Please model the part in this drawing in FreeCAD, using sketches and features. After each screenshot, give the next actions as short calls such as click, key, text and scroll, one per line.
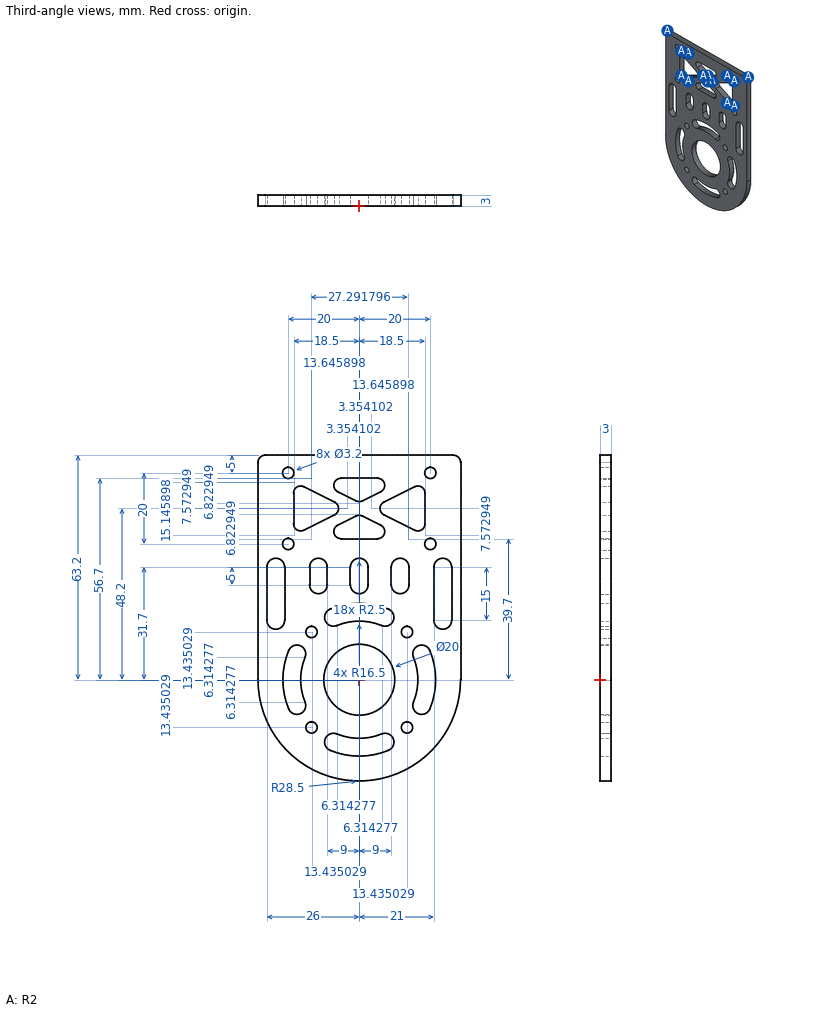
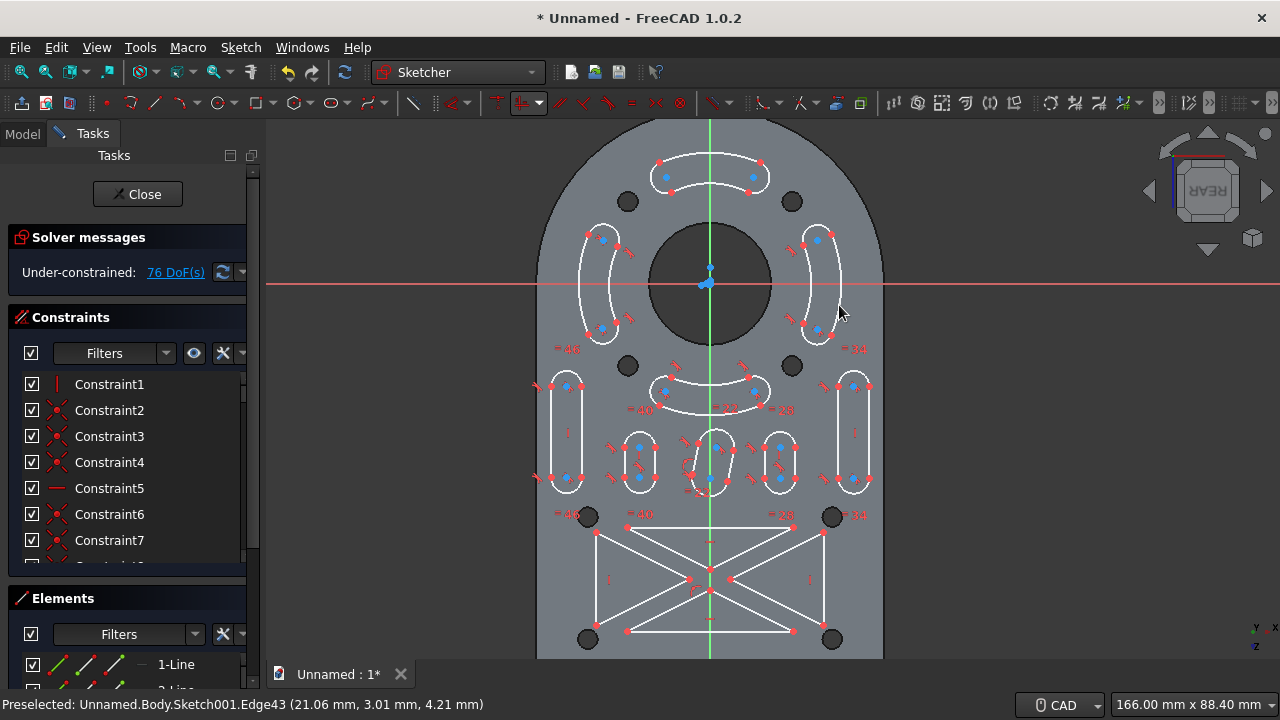
click(839, 305)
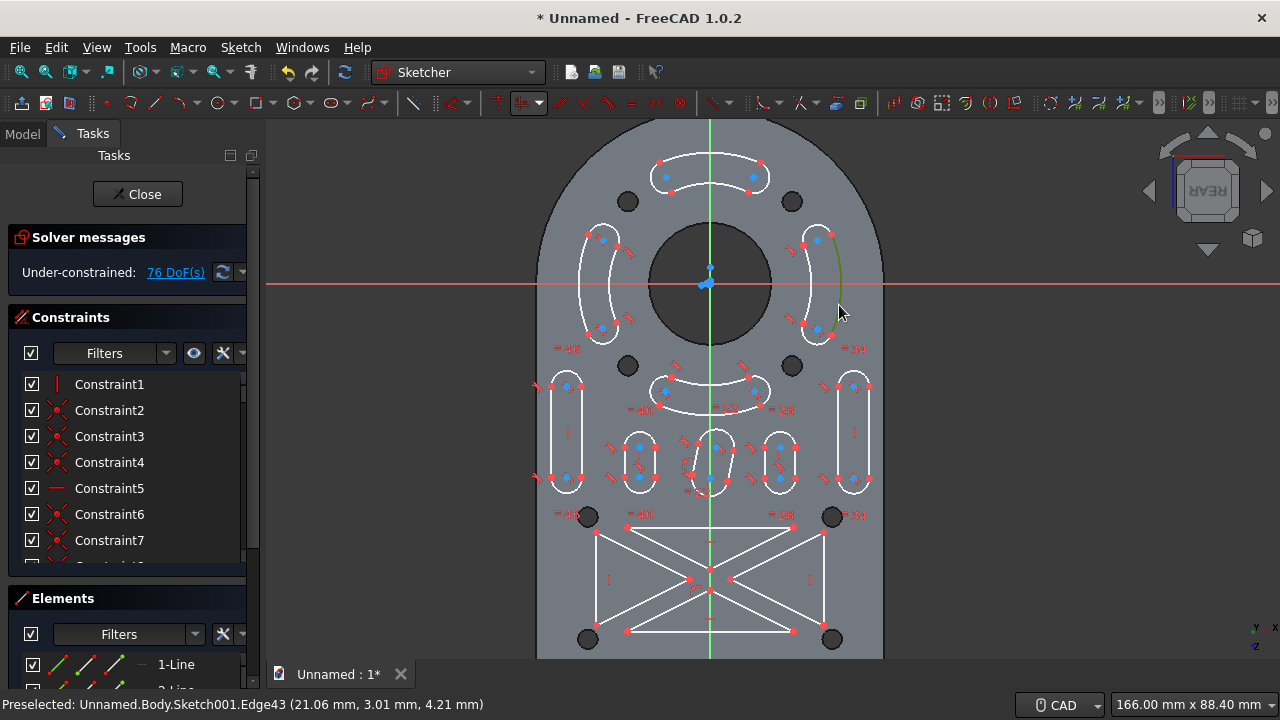
click(821, 225)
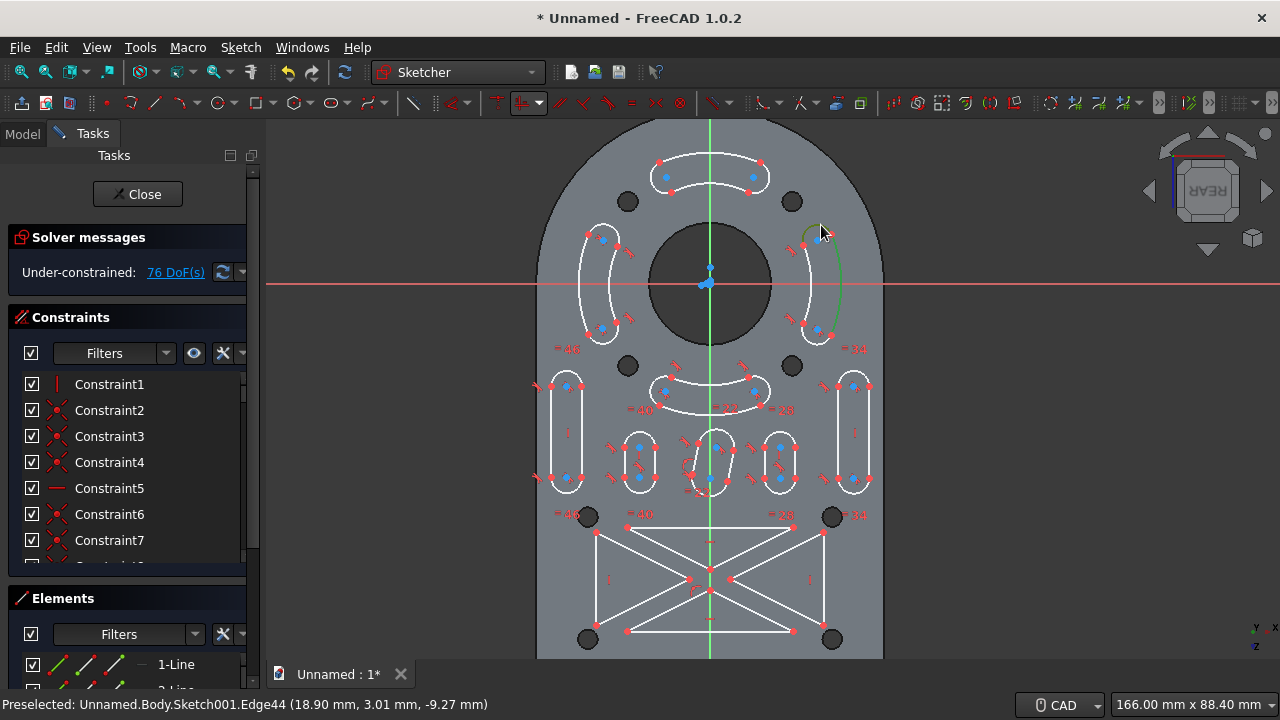
key(t)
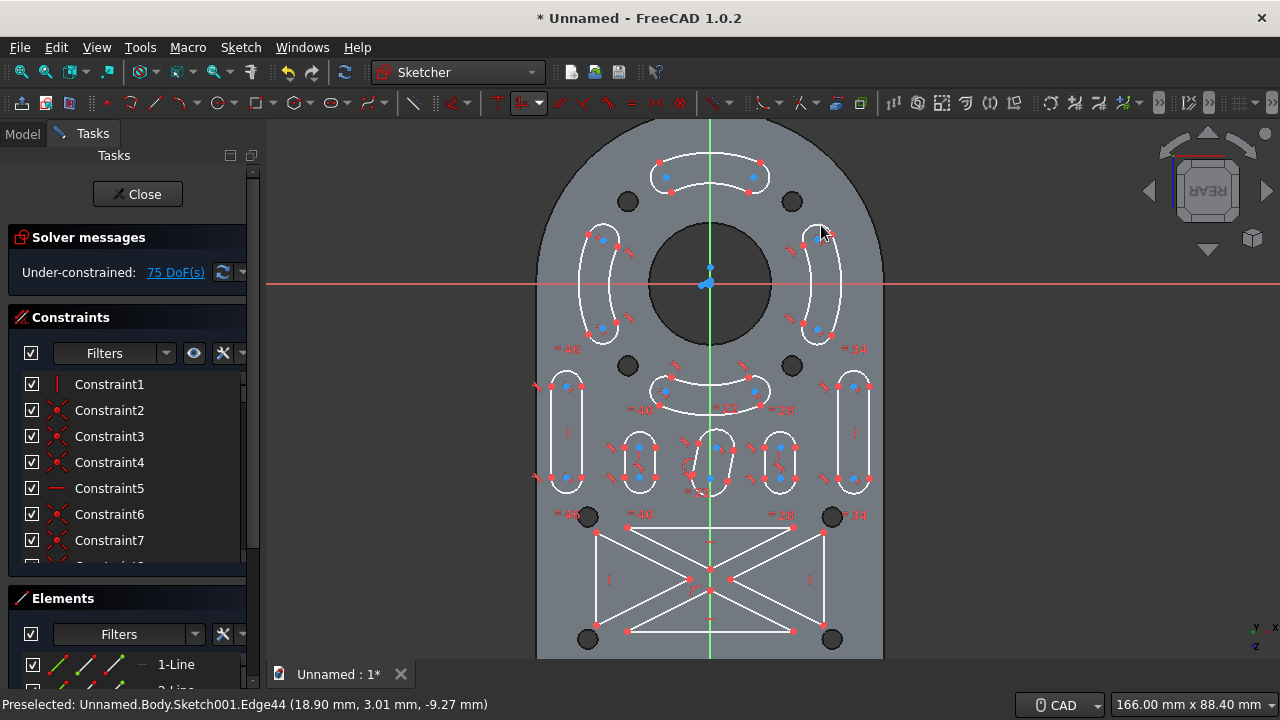
click(726, 185)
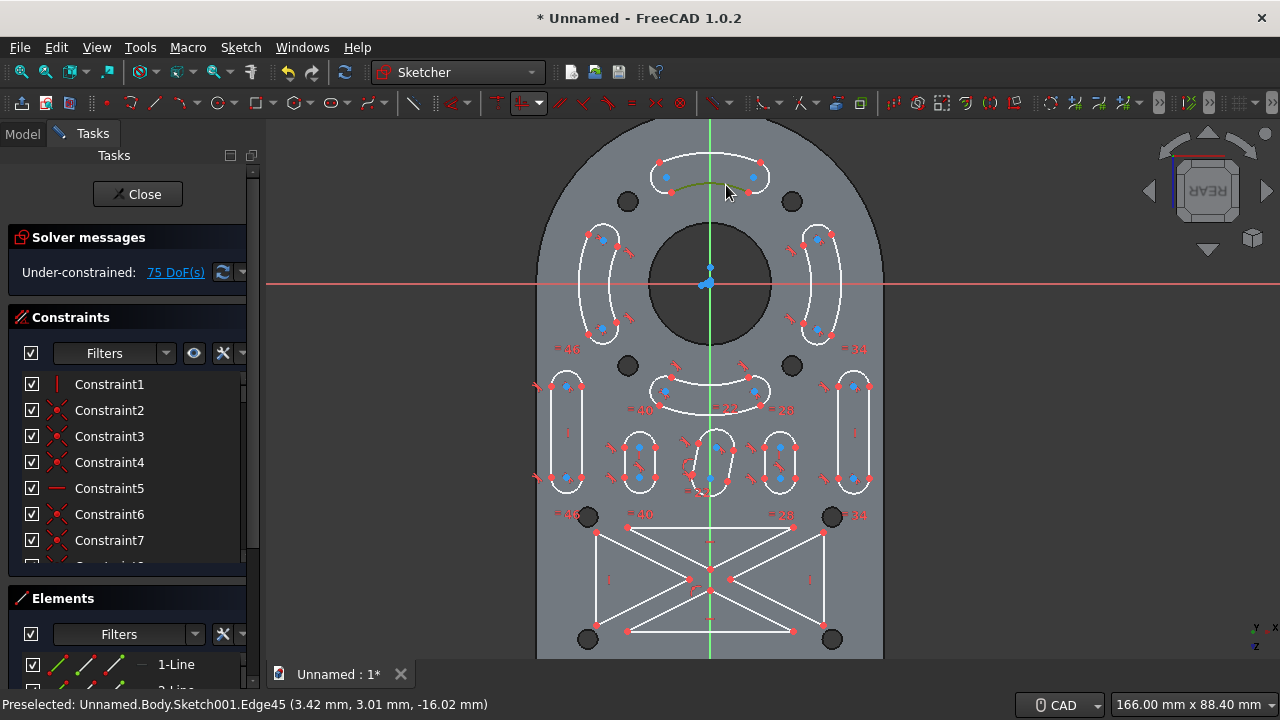
click(763, 190)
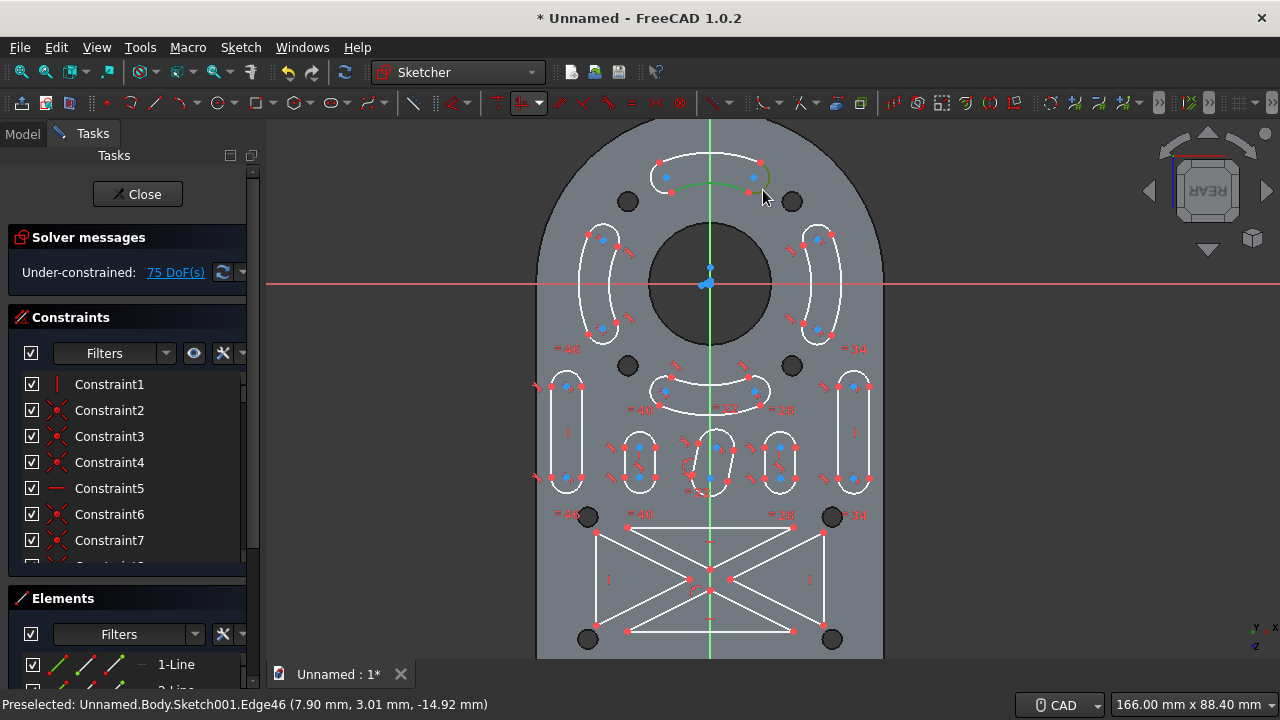
click(608, 104)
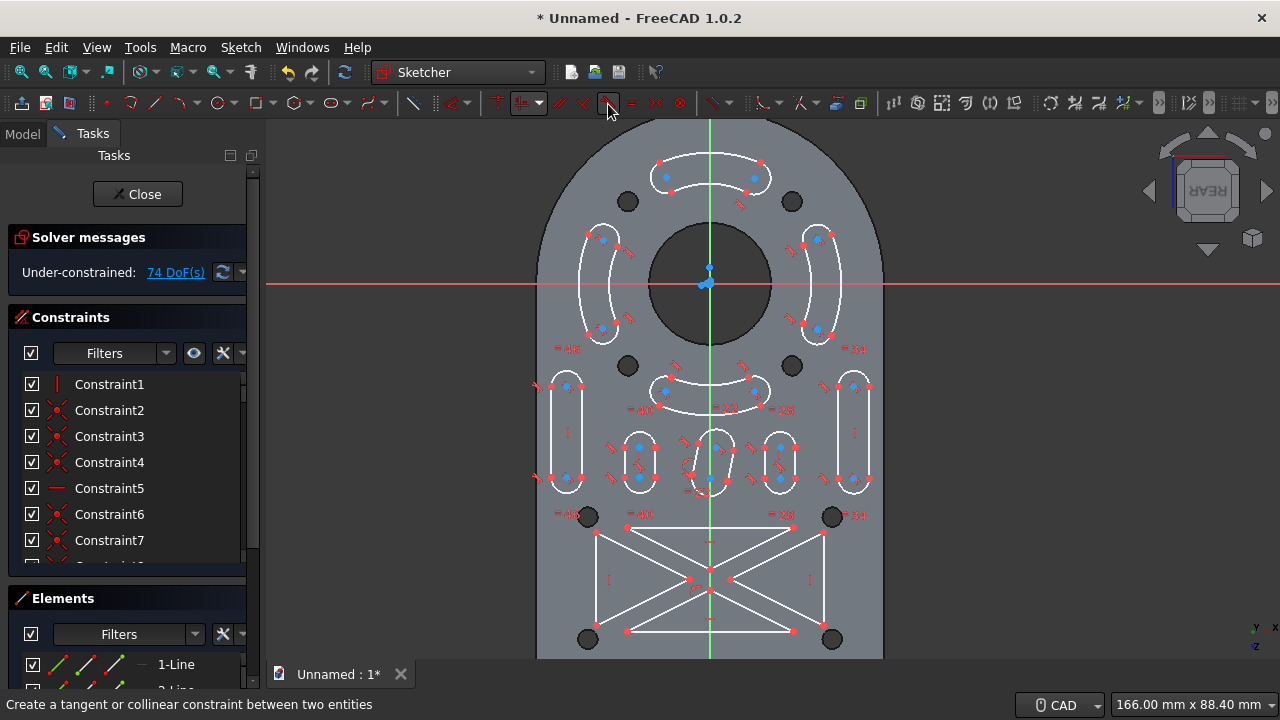
click(725, 185)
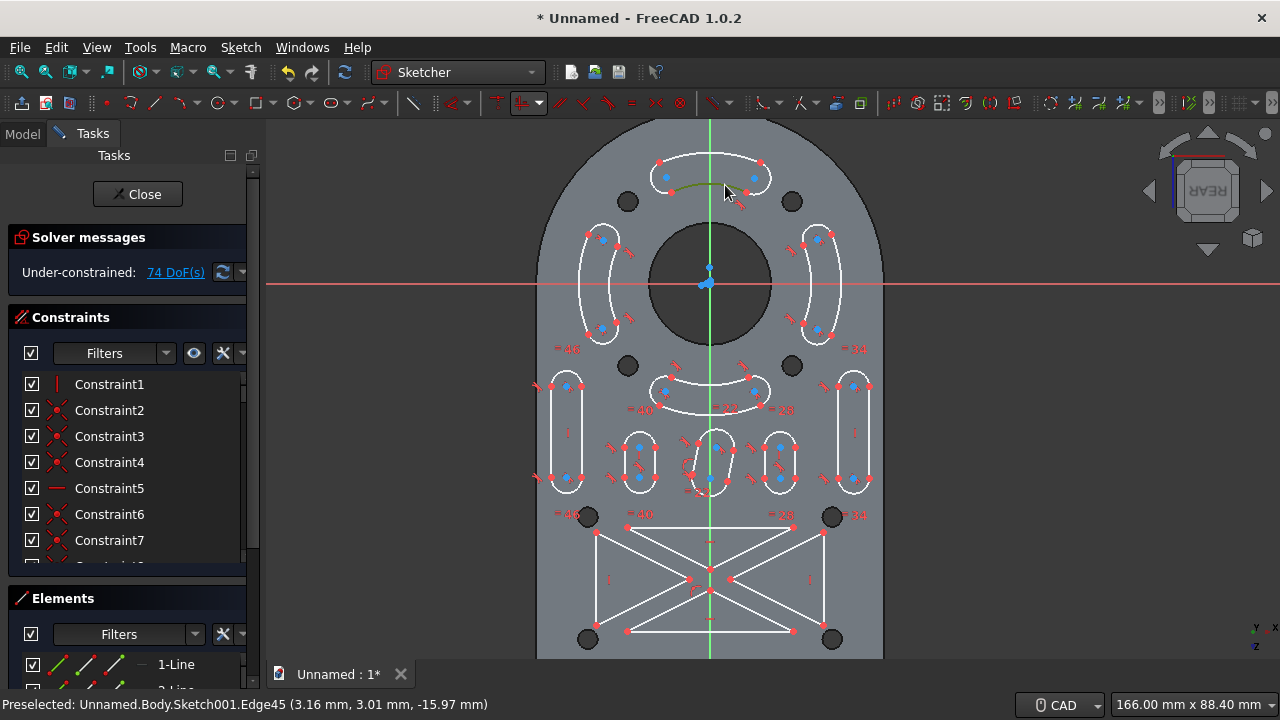
click(651, 174)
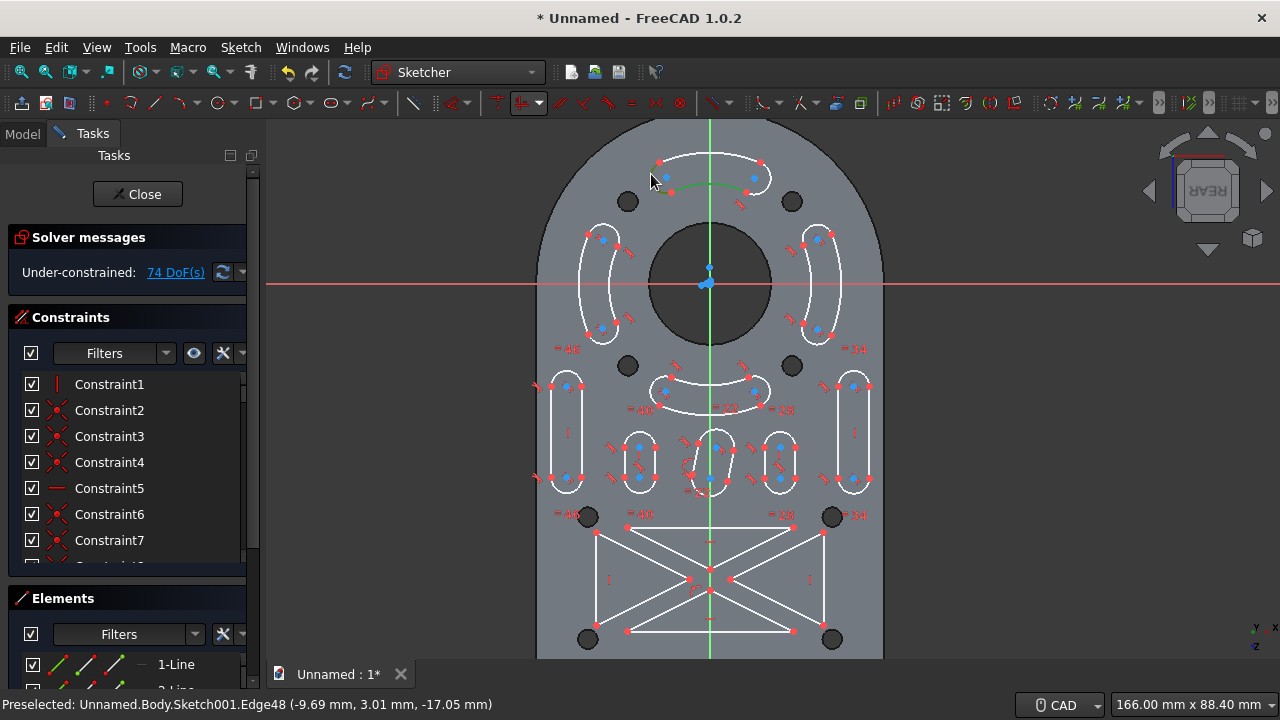
click(608, 104)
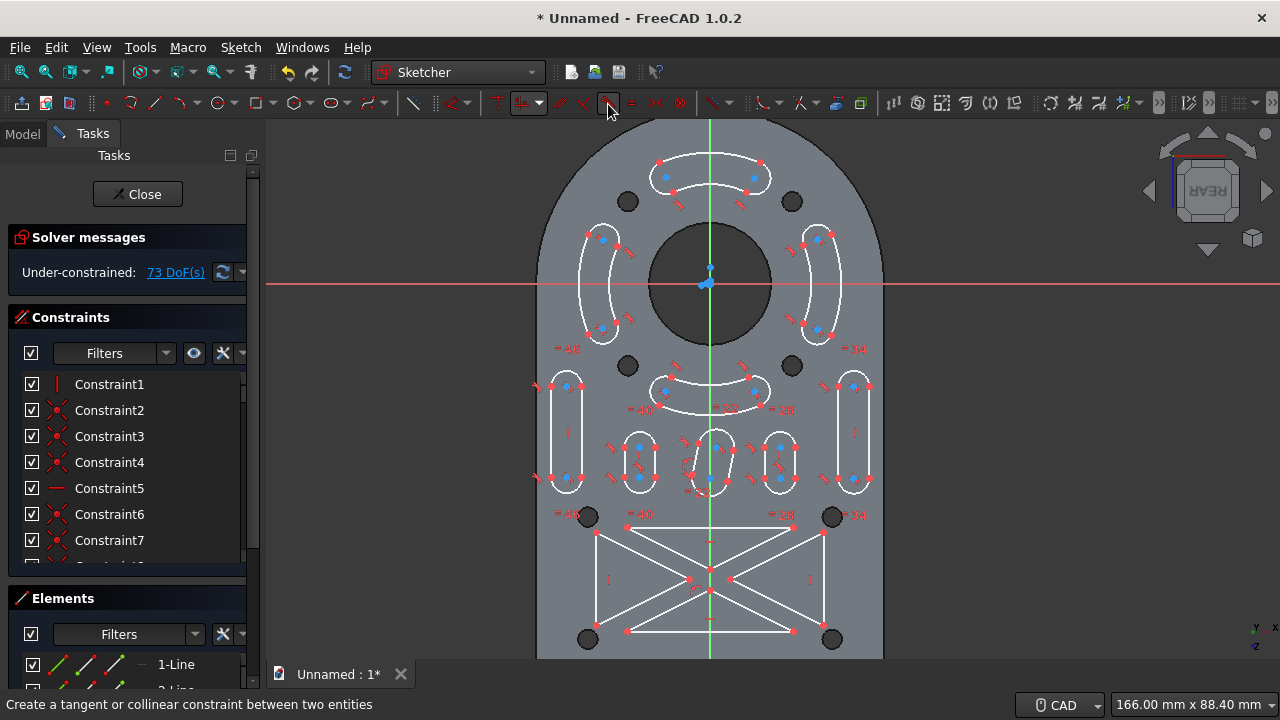
click(762, 192)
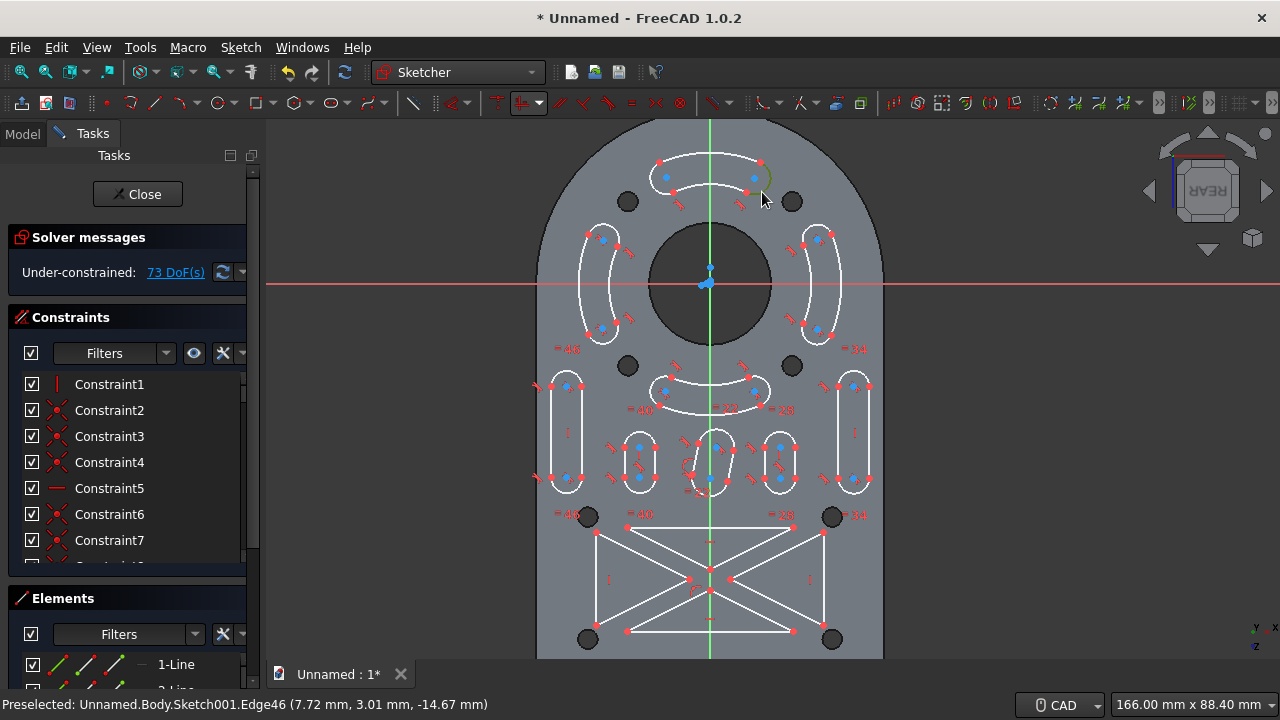
click(731, 154)